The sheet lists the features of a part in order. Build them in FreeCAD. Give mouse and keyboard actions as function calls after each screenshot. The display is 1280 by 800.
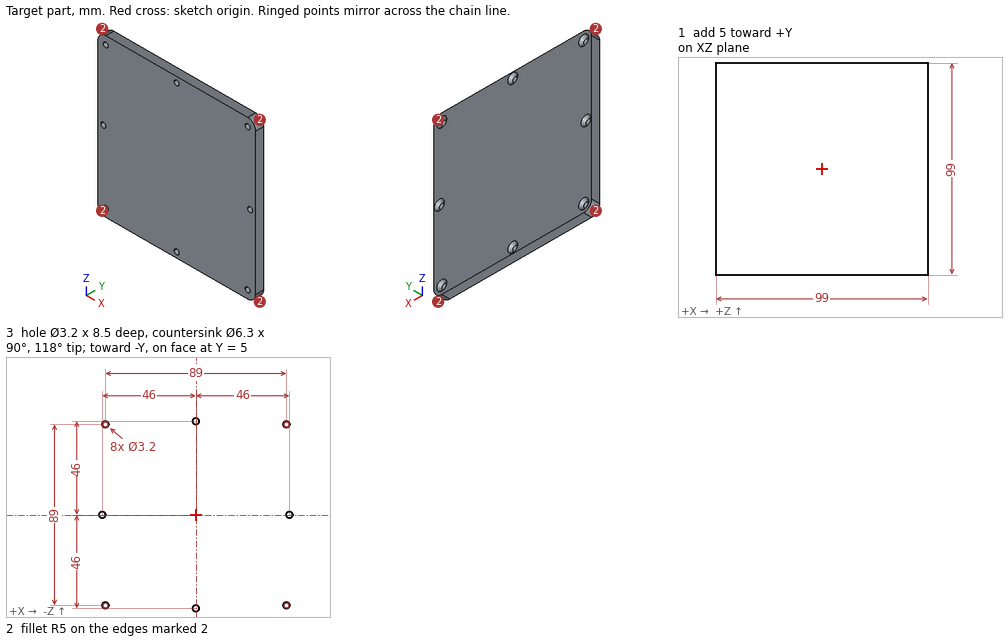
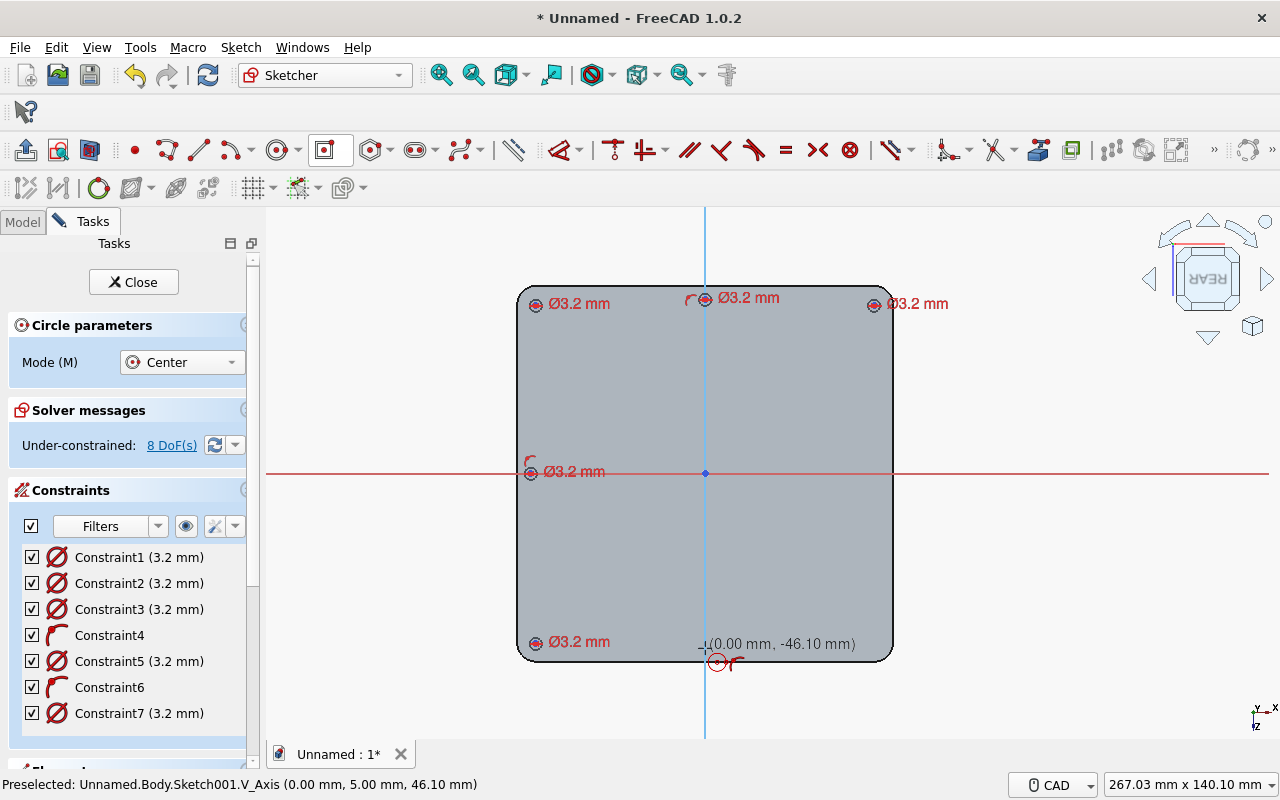
click(705, 648)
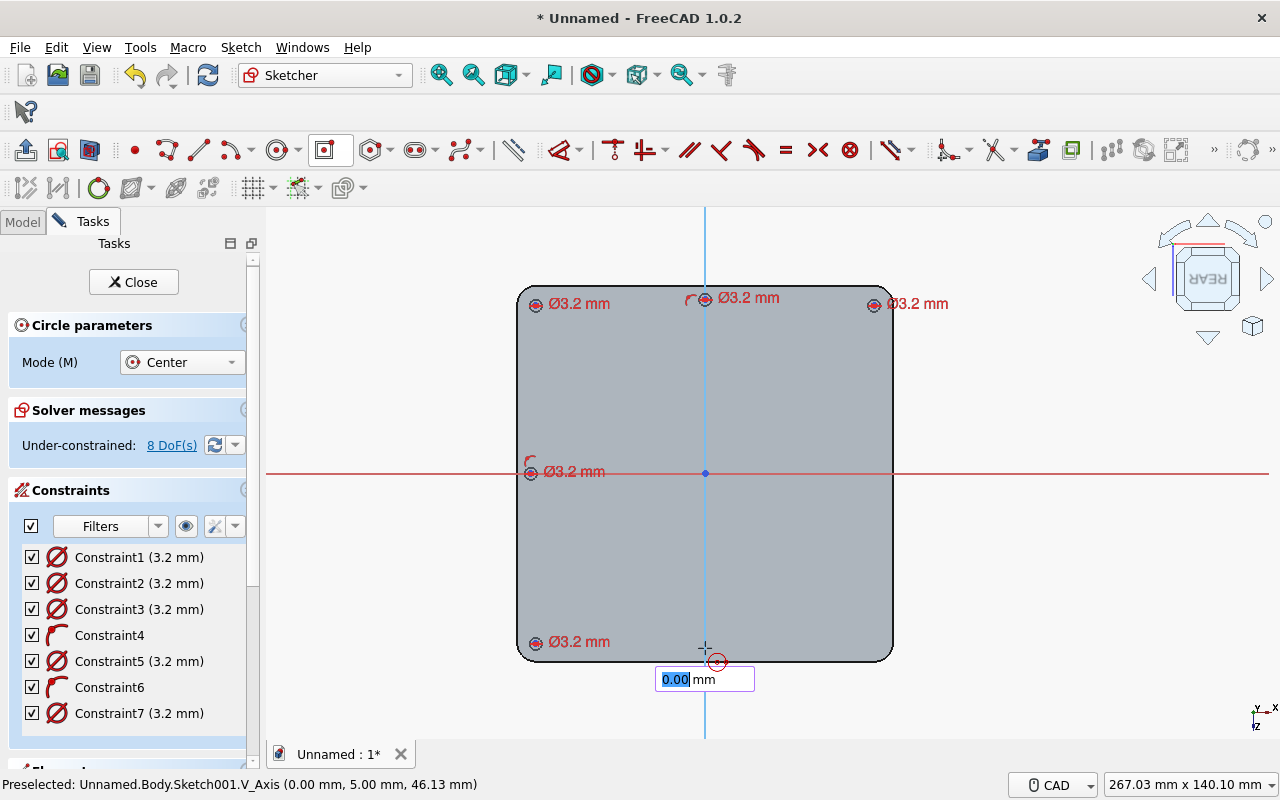
scroll(711, 646, up, 6)
move(709, 645)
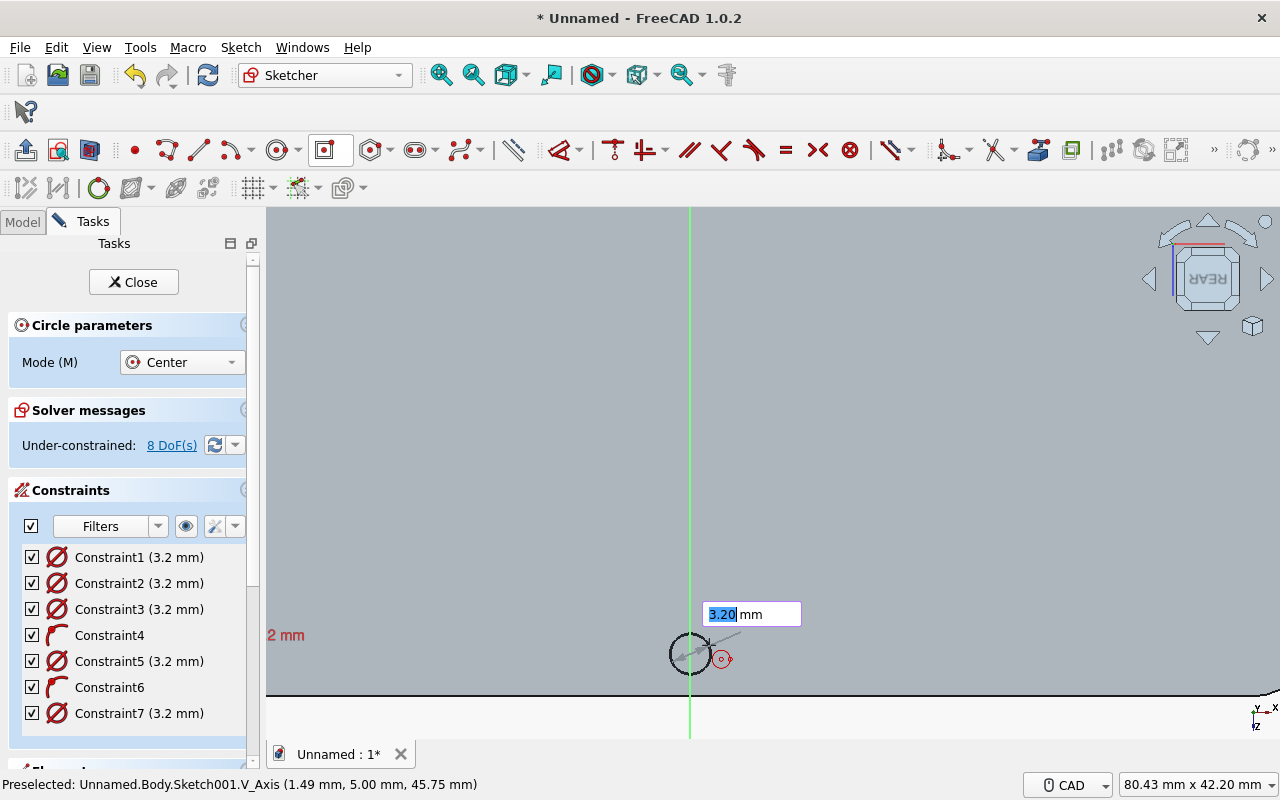
text(3.2)
key(Return)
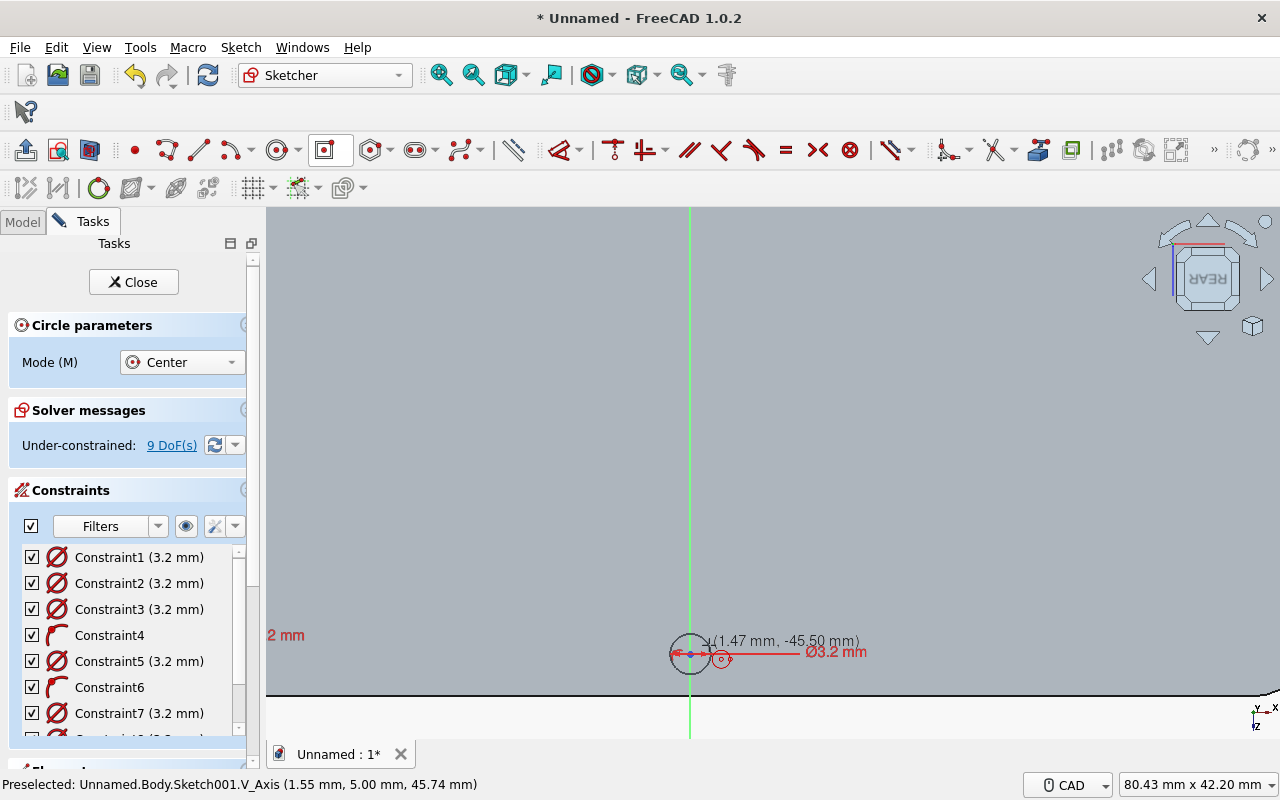
scroll(711, 646, down, 6)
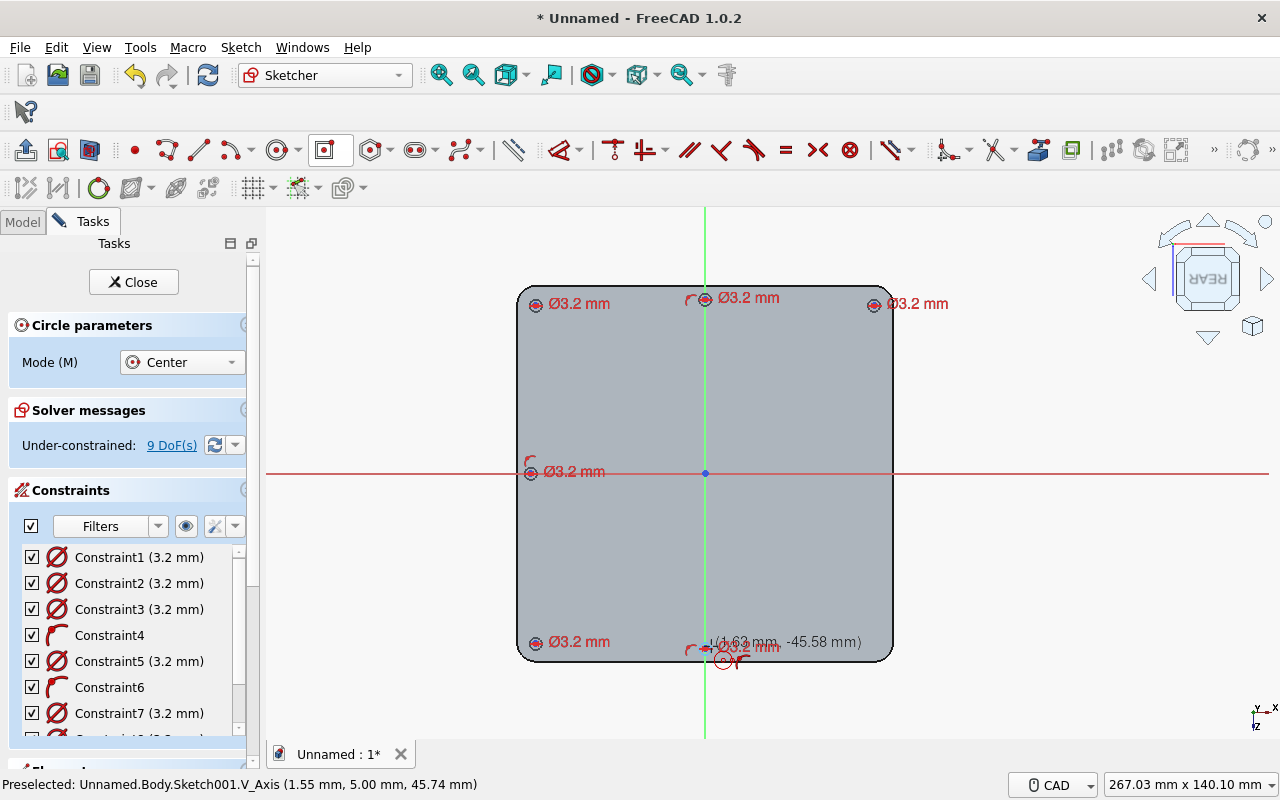
scroll(874, 643, up, 7)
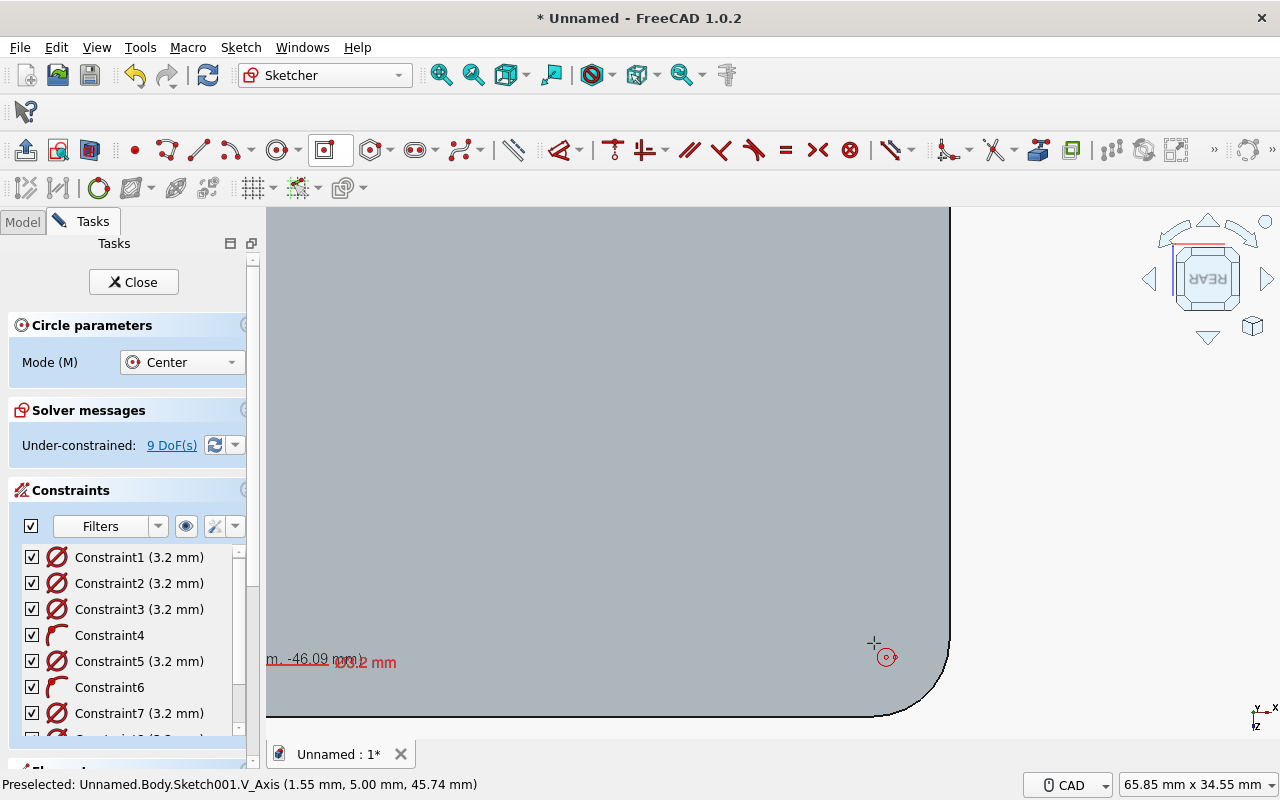
scroll(874, 643, down, 7)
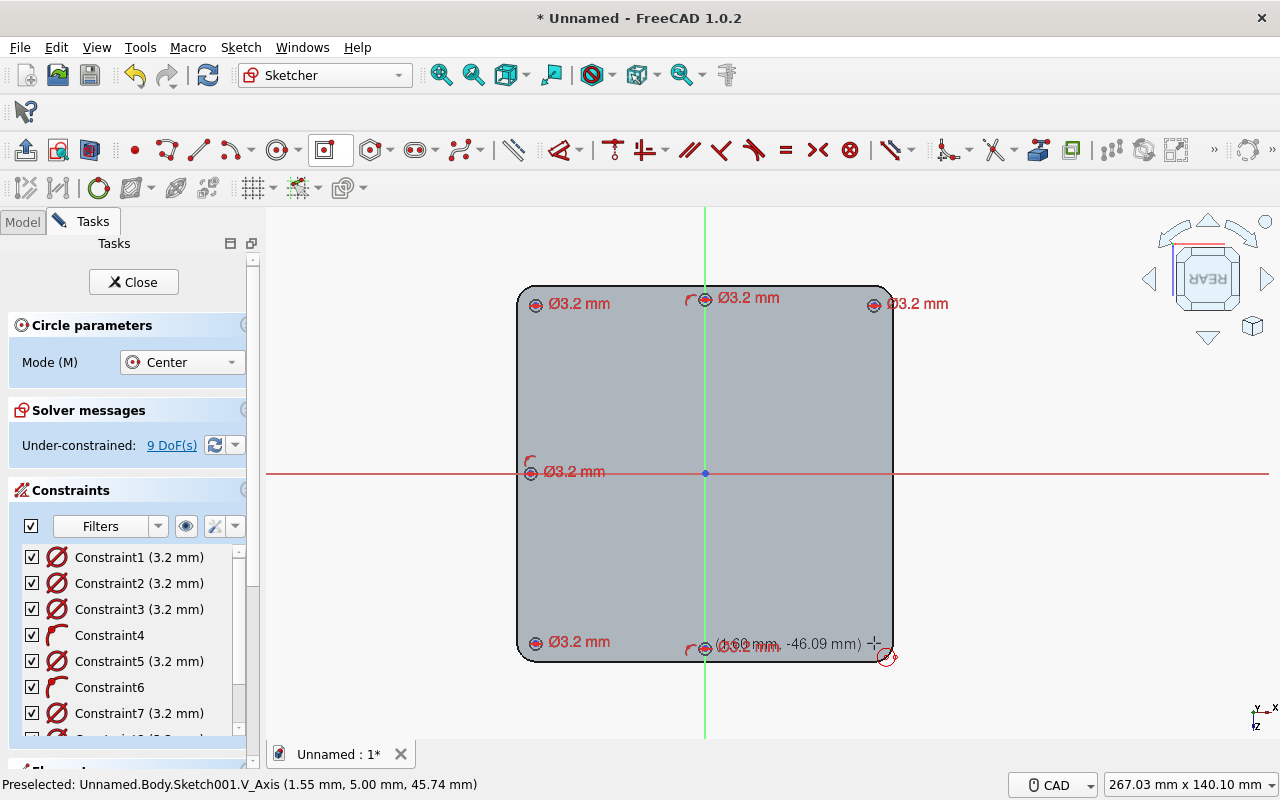
click(874, 643)
move(878, 638)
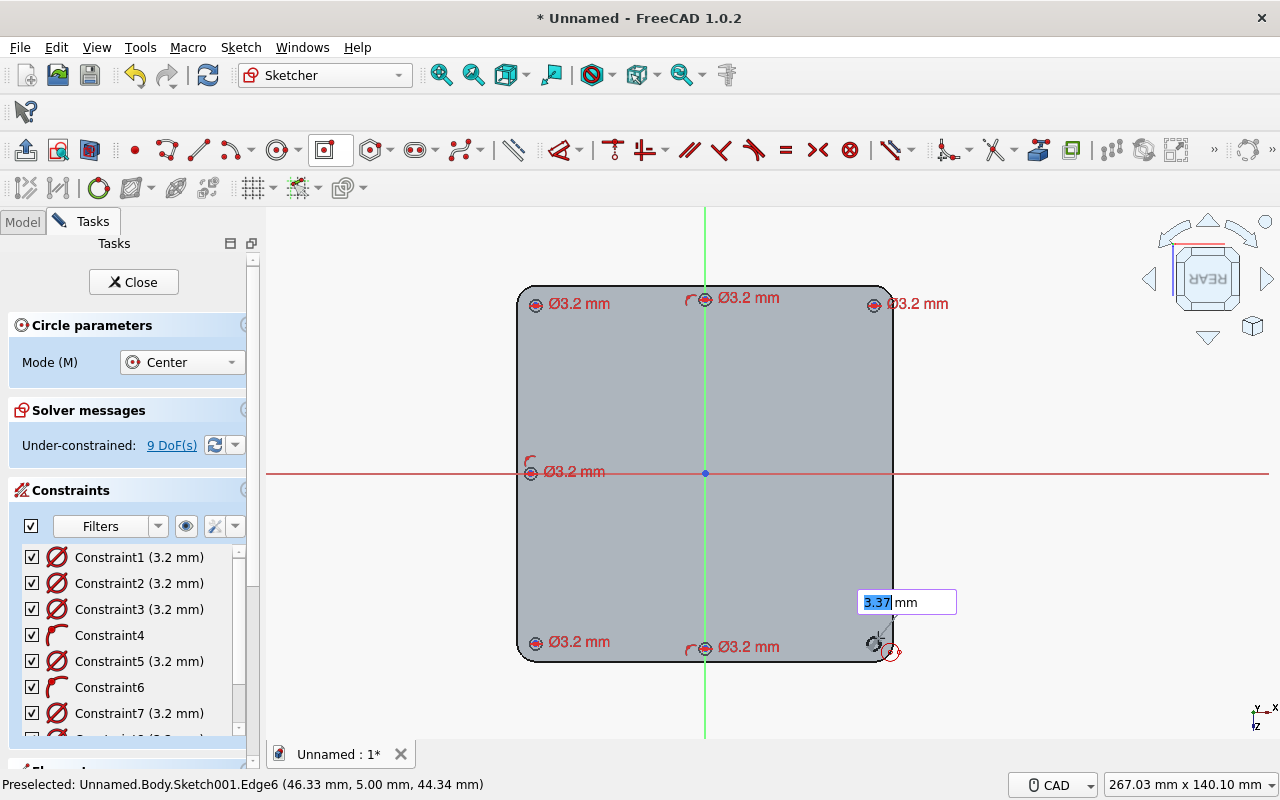
text(3.2)
key(Return)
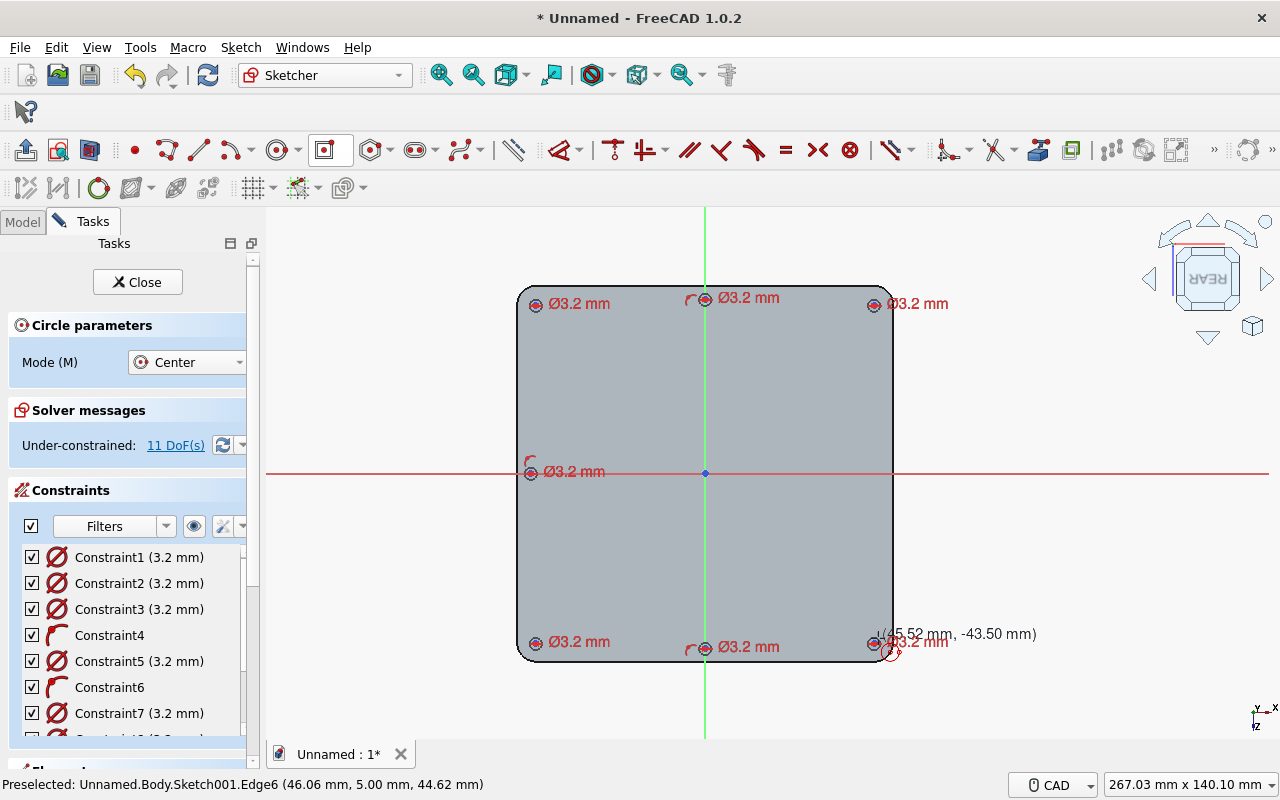
scroll(880, 474, up, 7)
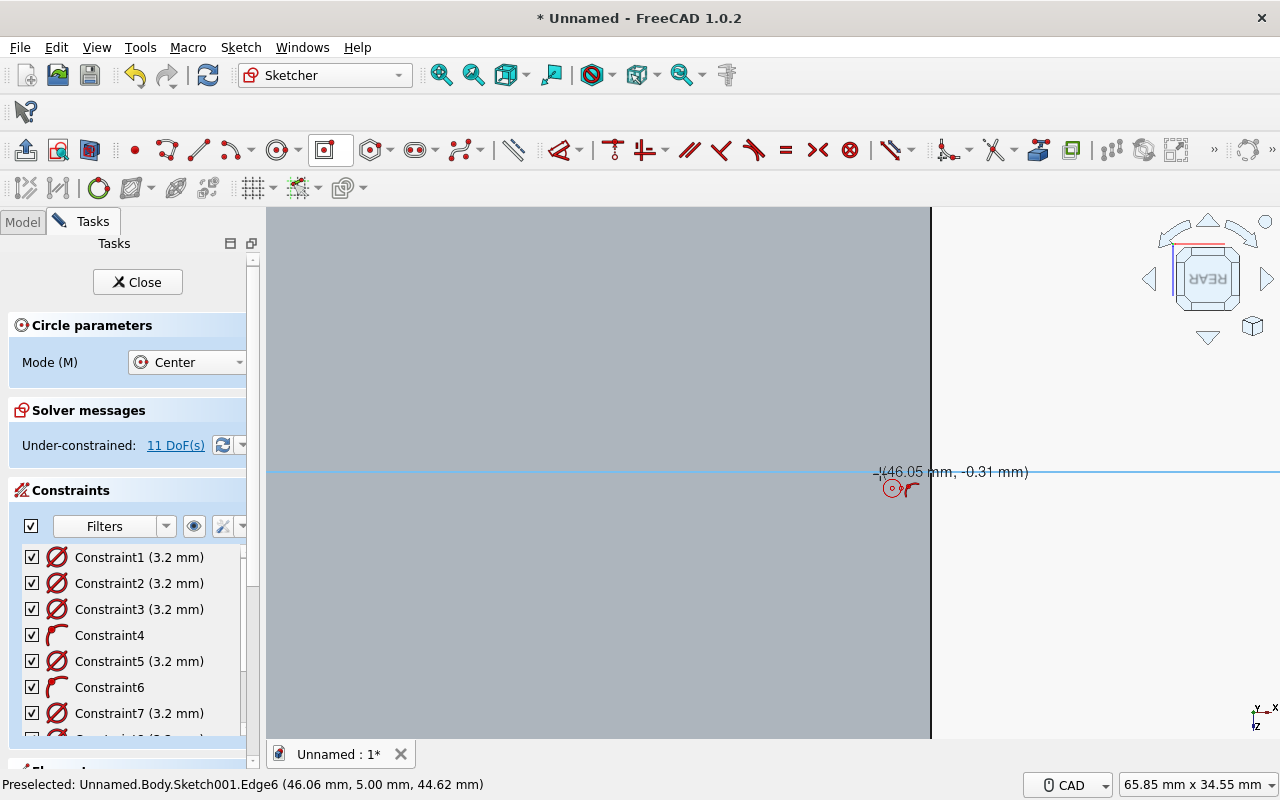
scroll(880, 473, down, 7)